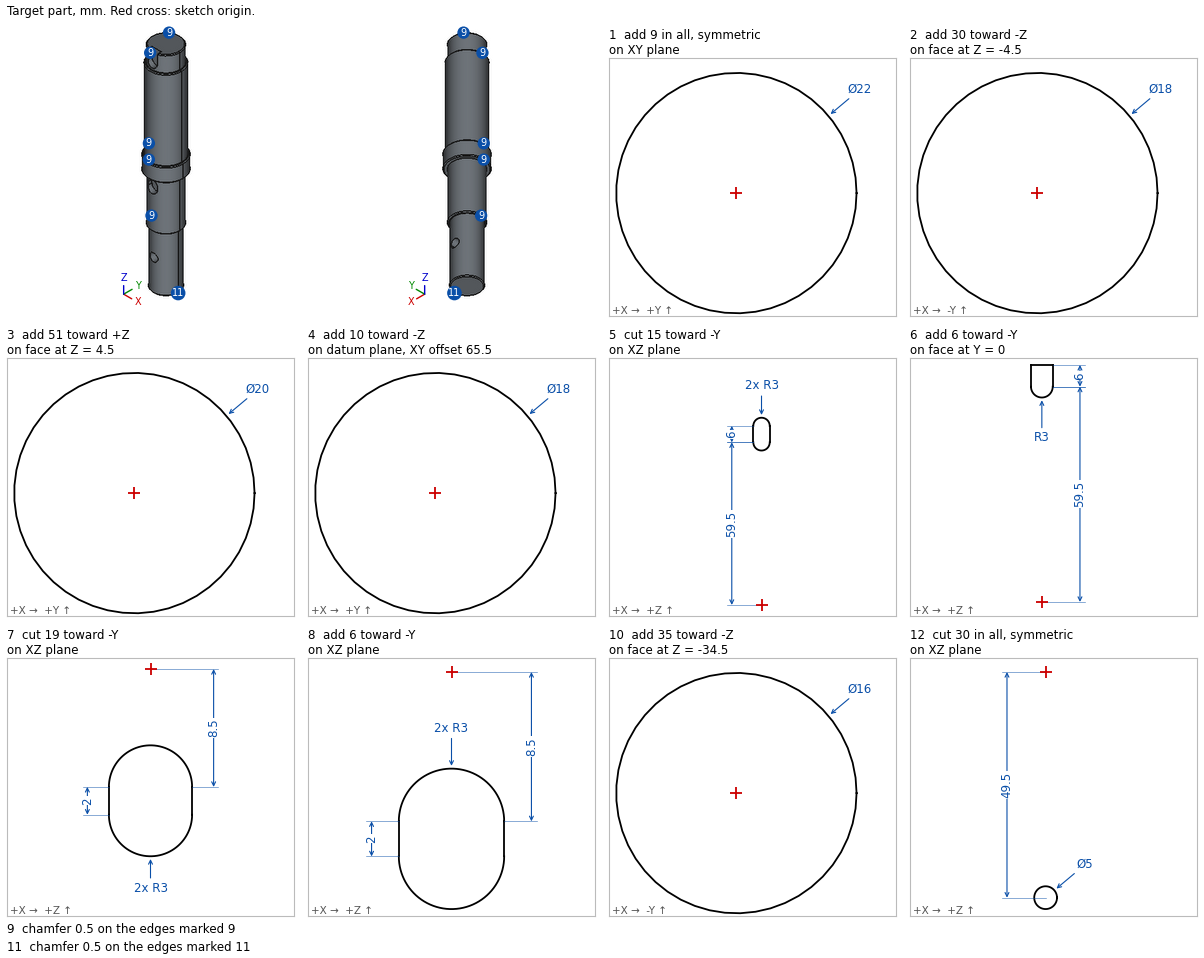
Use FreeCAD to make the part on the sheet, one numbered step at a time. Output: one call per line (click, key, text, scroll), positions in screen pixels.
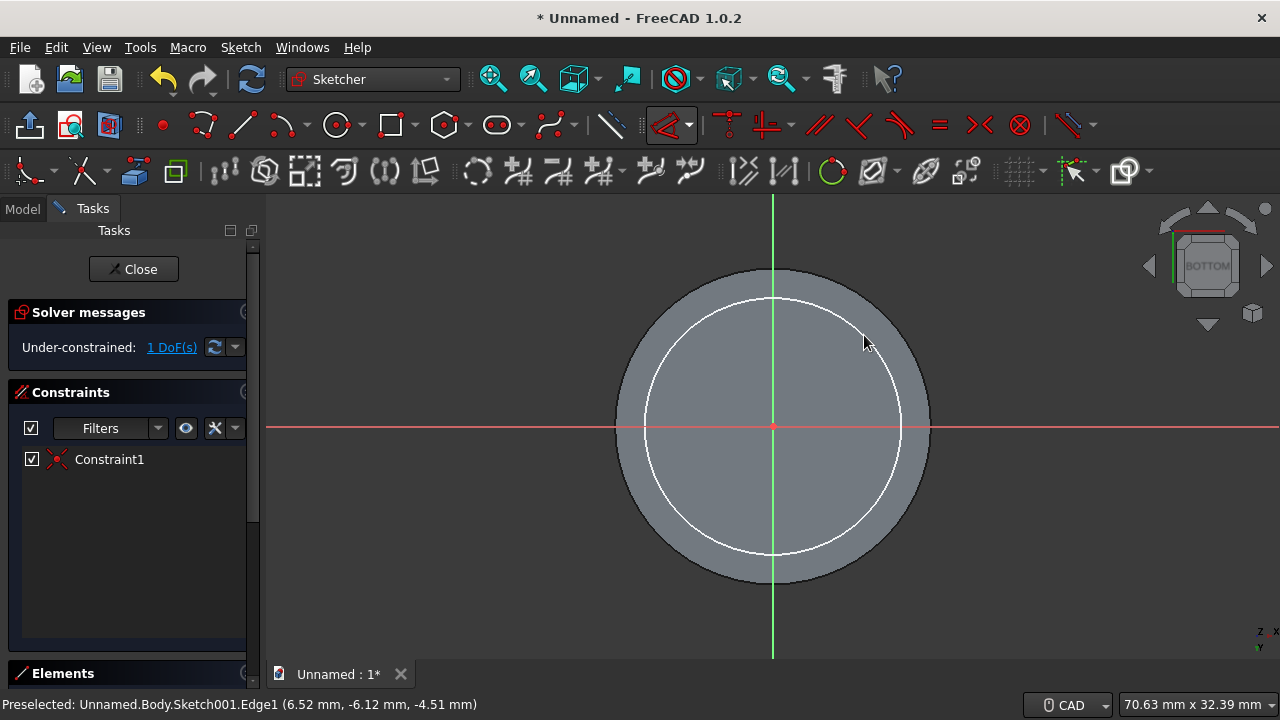
click(863, 335)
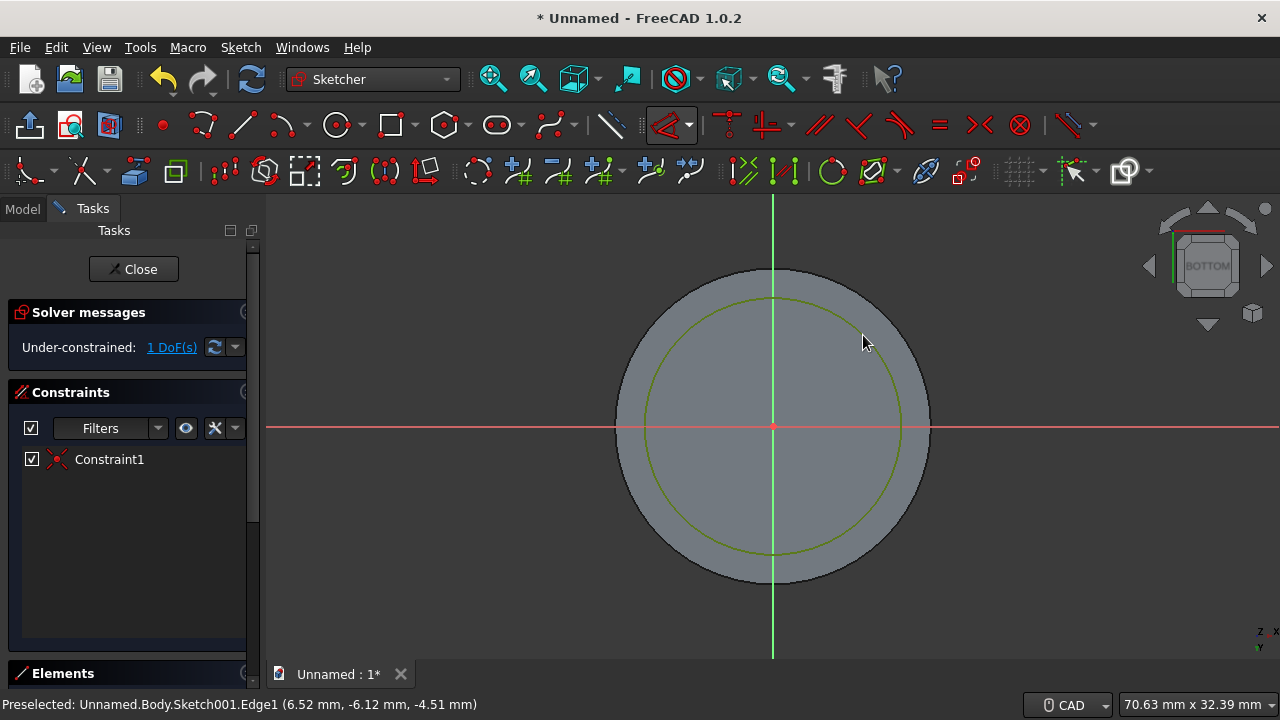
click(692, 126)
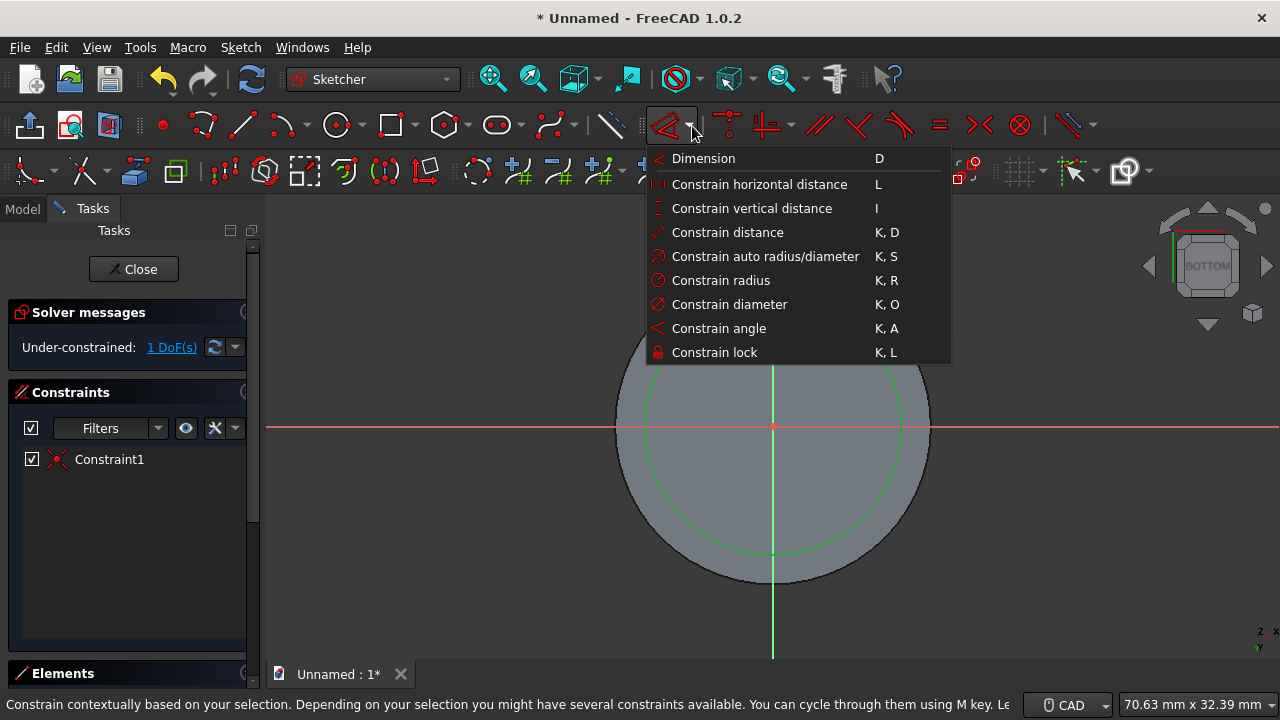
click(799, 304)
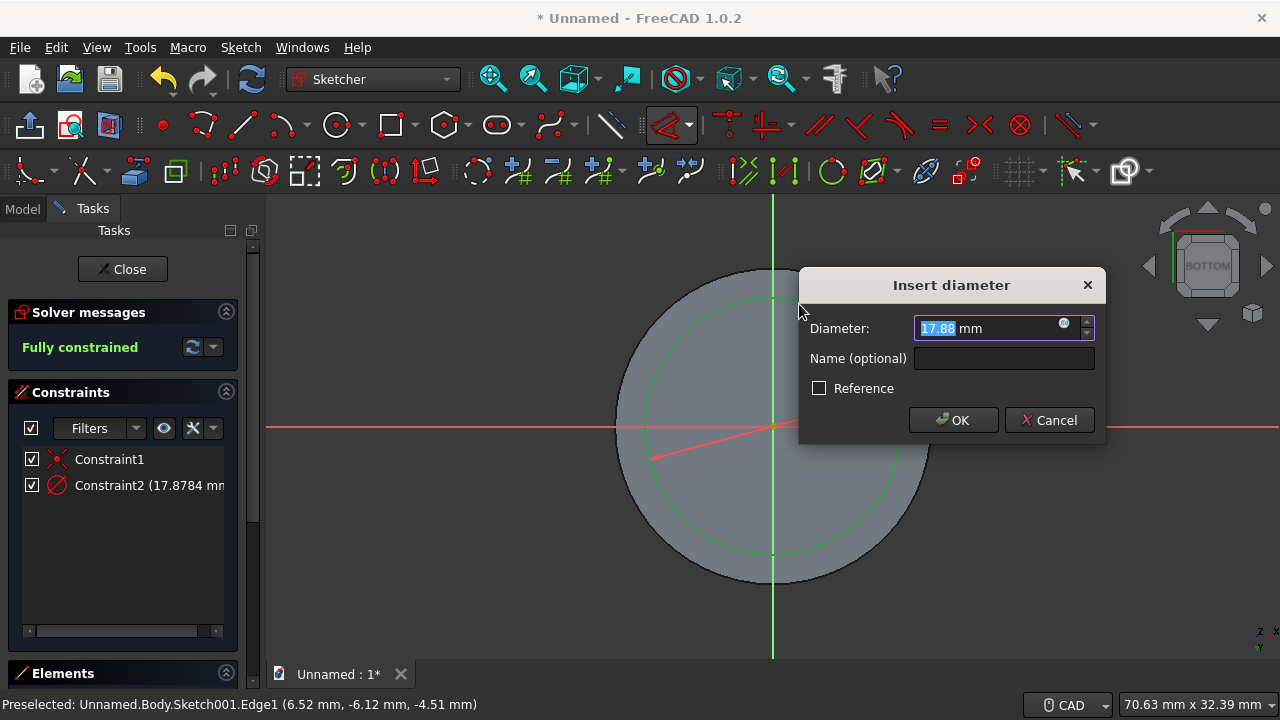
text(18)
key(Return)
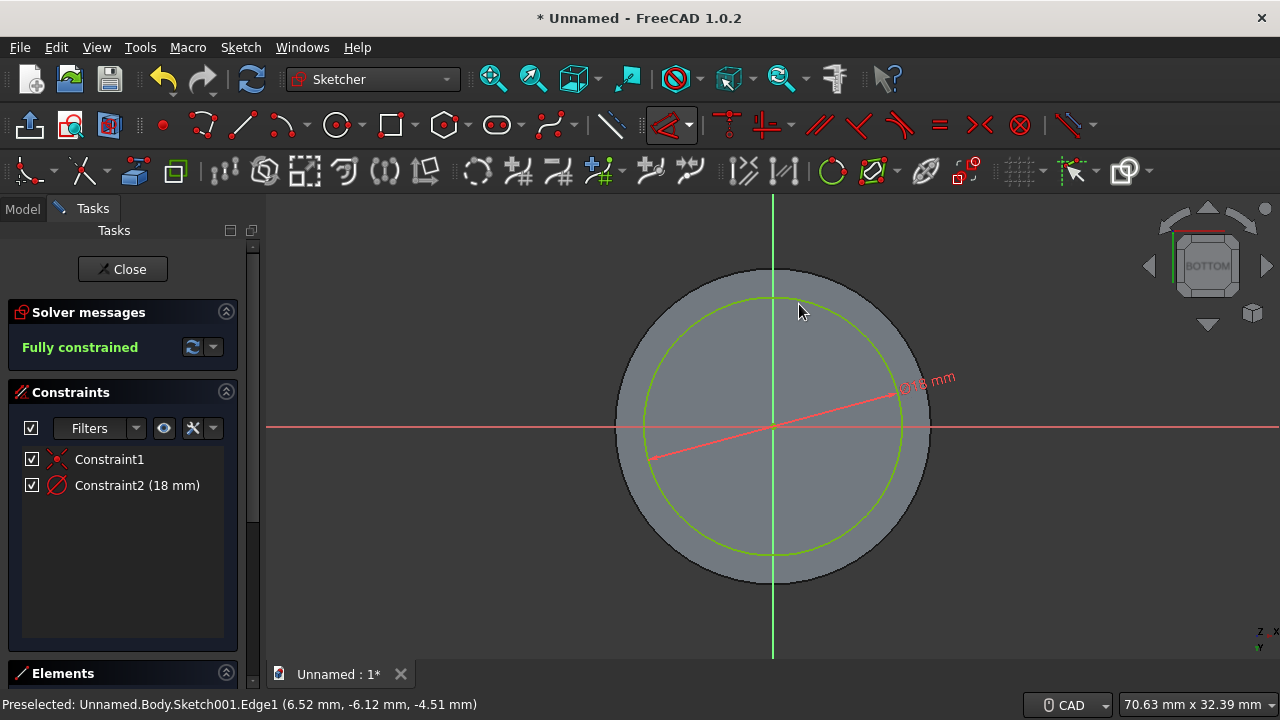
click(123, 269)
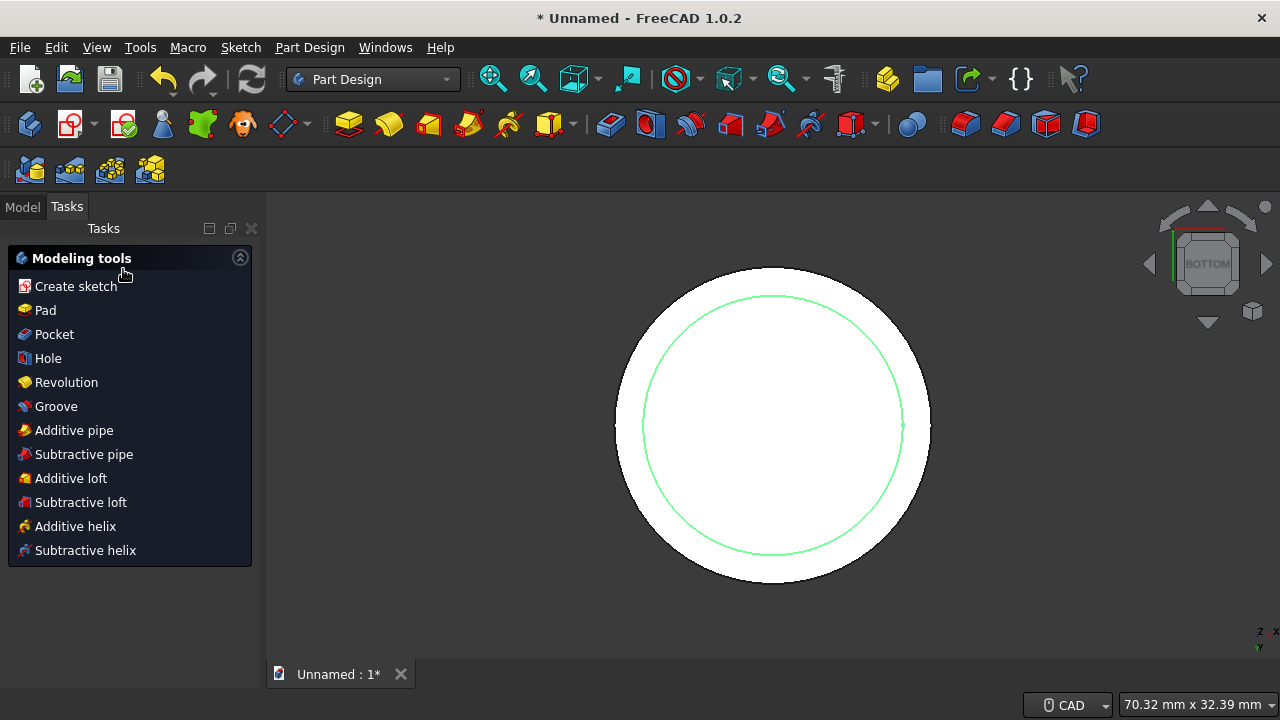
click(350, 124)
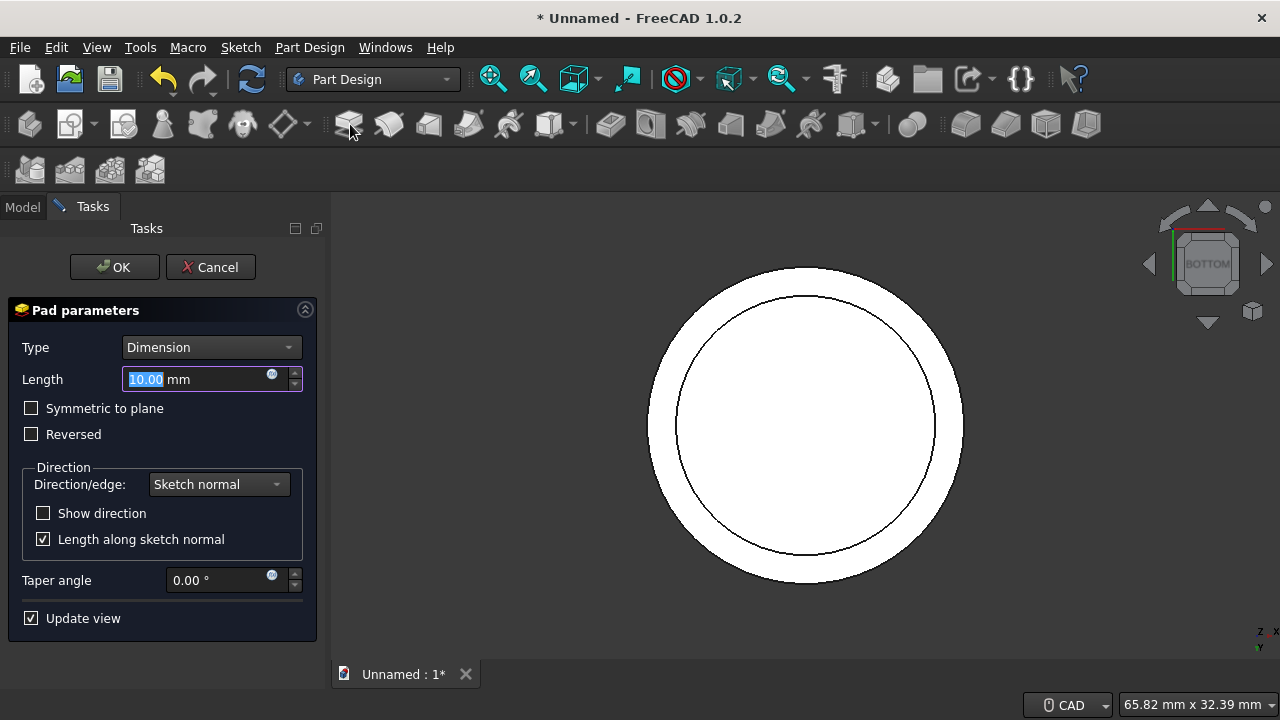
text(30)
key(Tab)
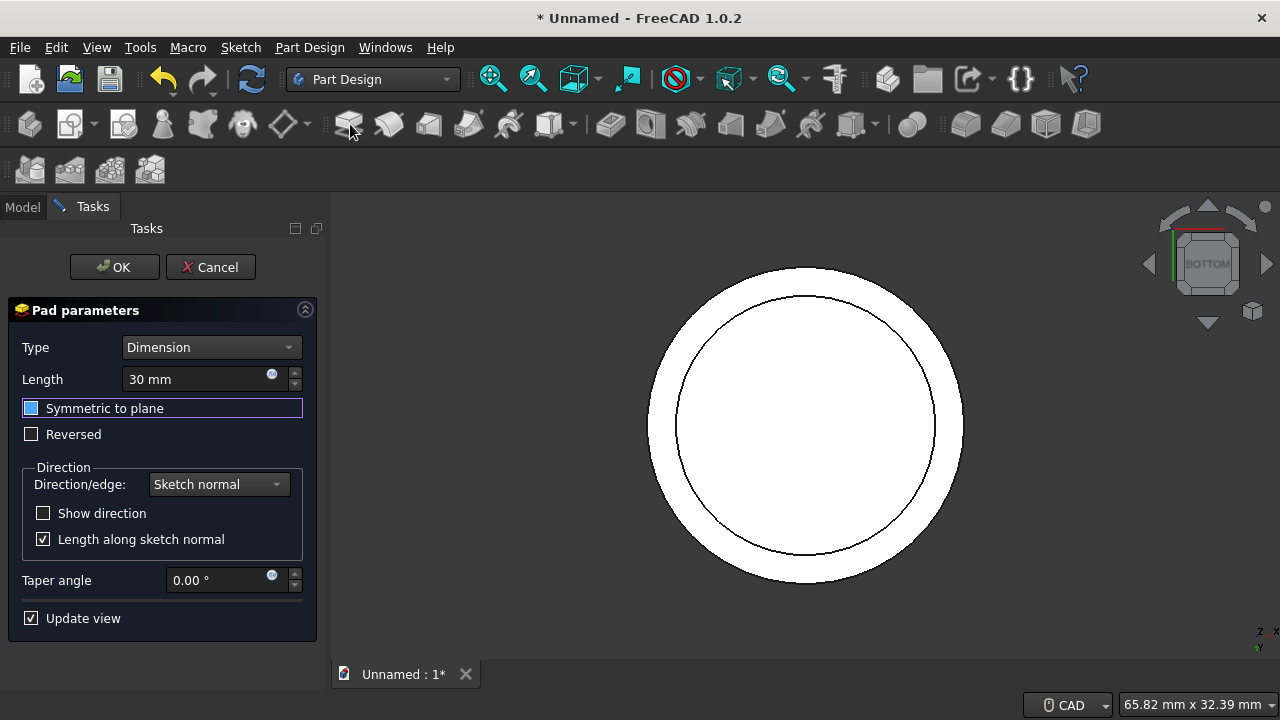
click(115, 267)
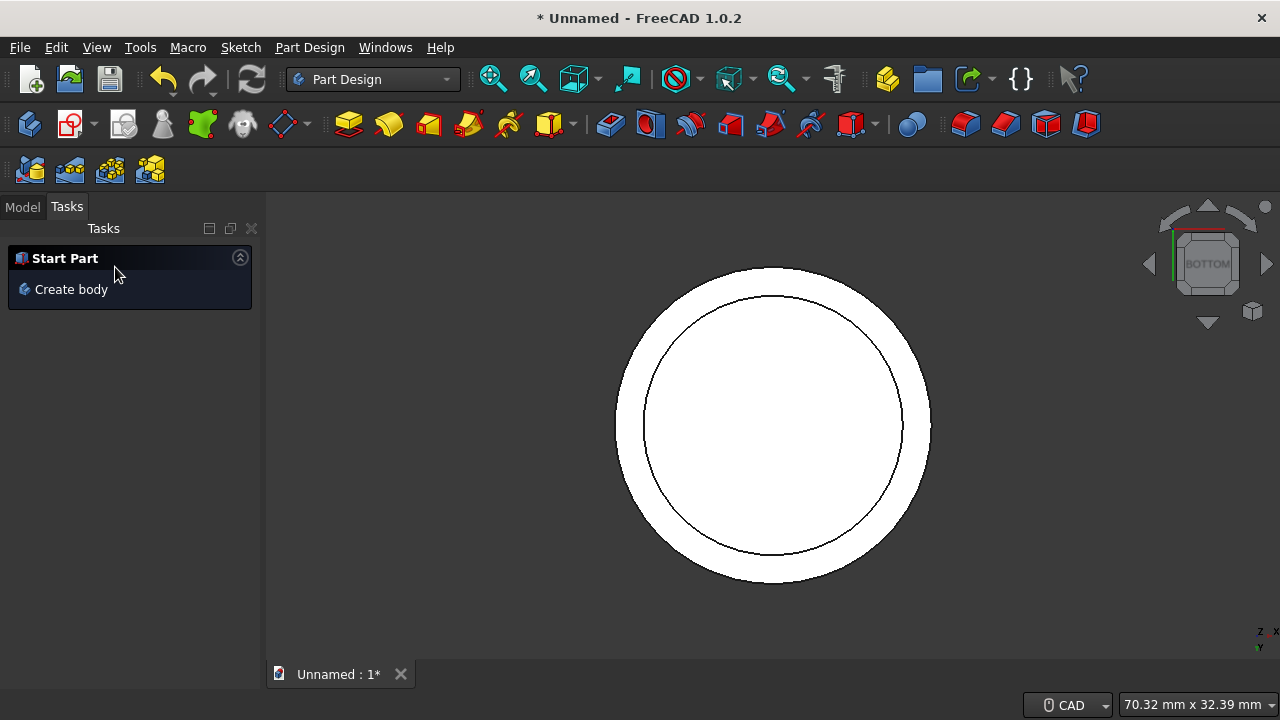
key(0)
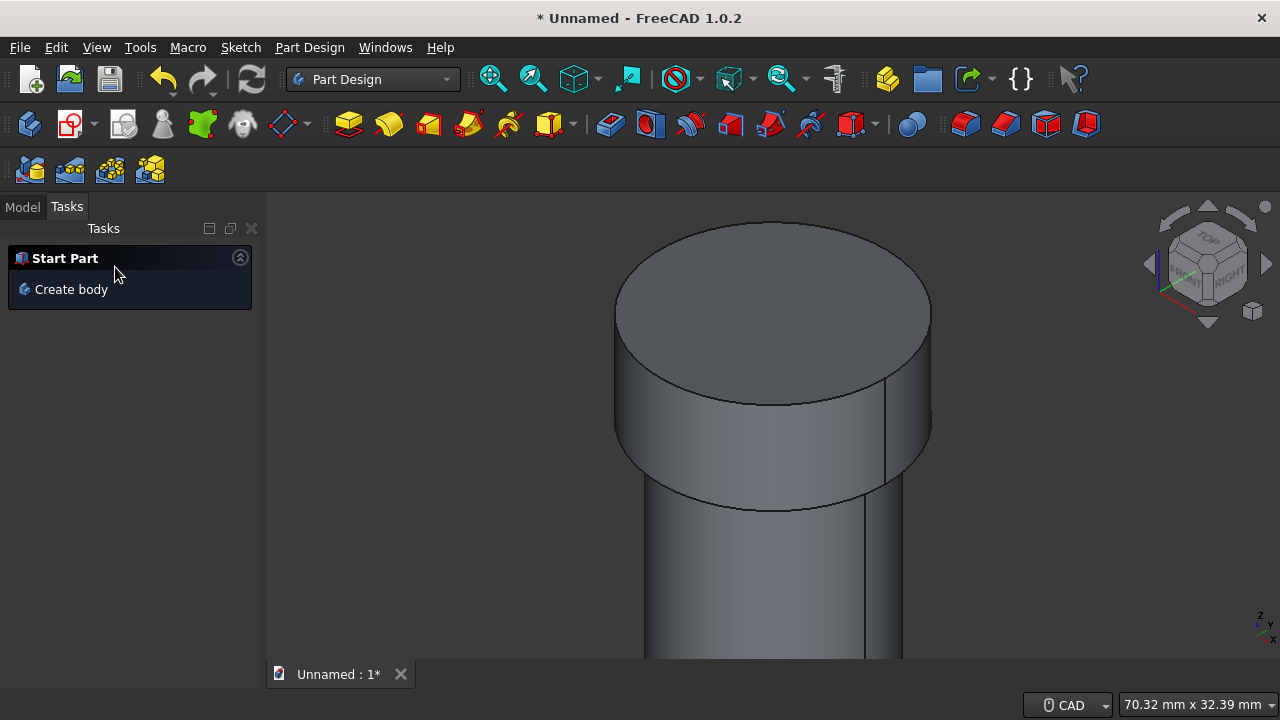
click(494, 80)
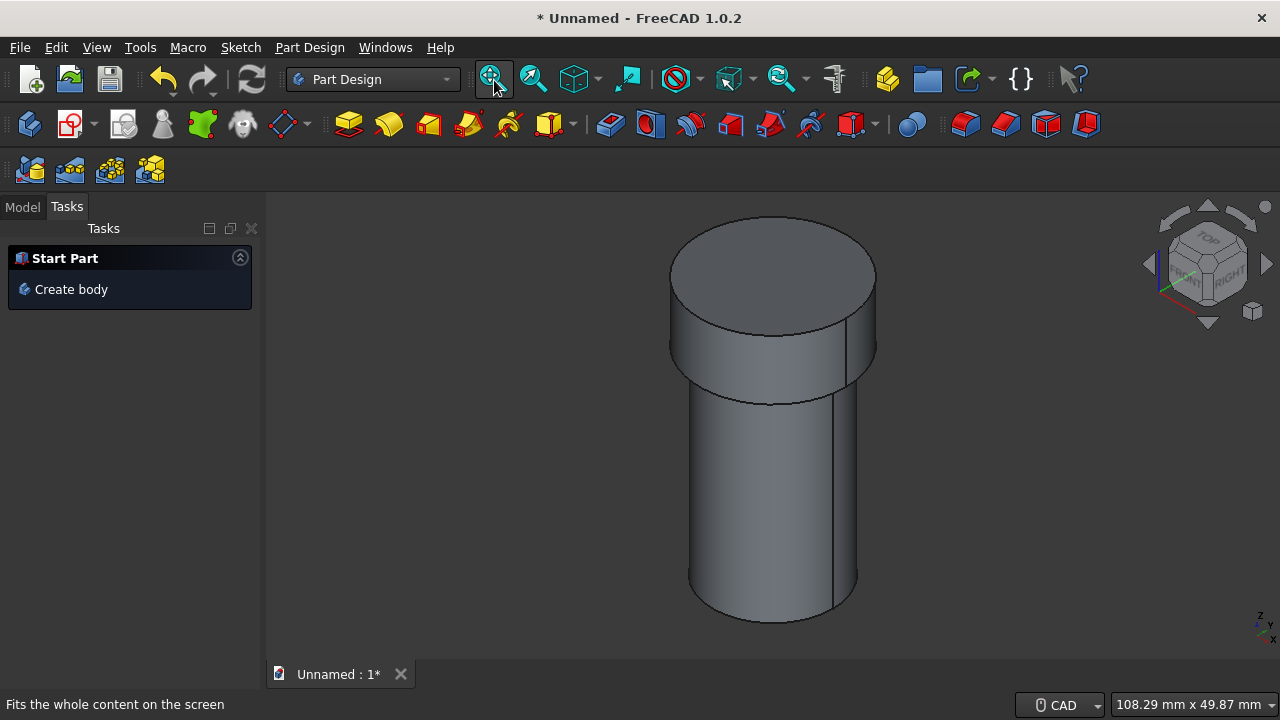
click(773, 275)